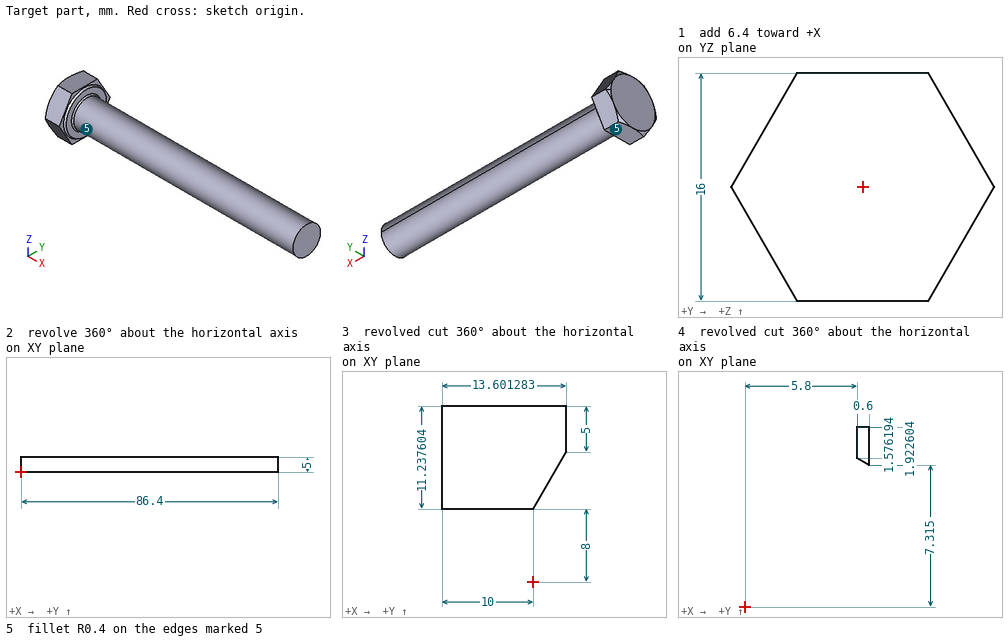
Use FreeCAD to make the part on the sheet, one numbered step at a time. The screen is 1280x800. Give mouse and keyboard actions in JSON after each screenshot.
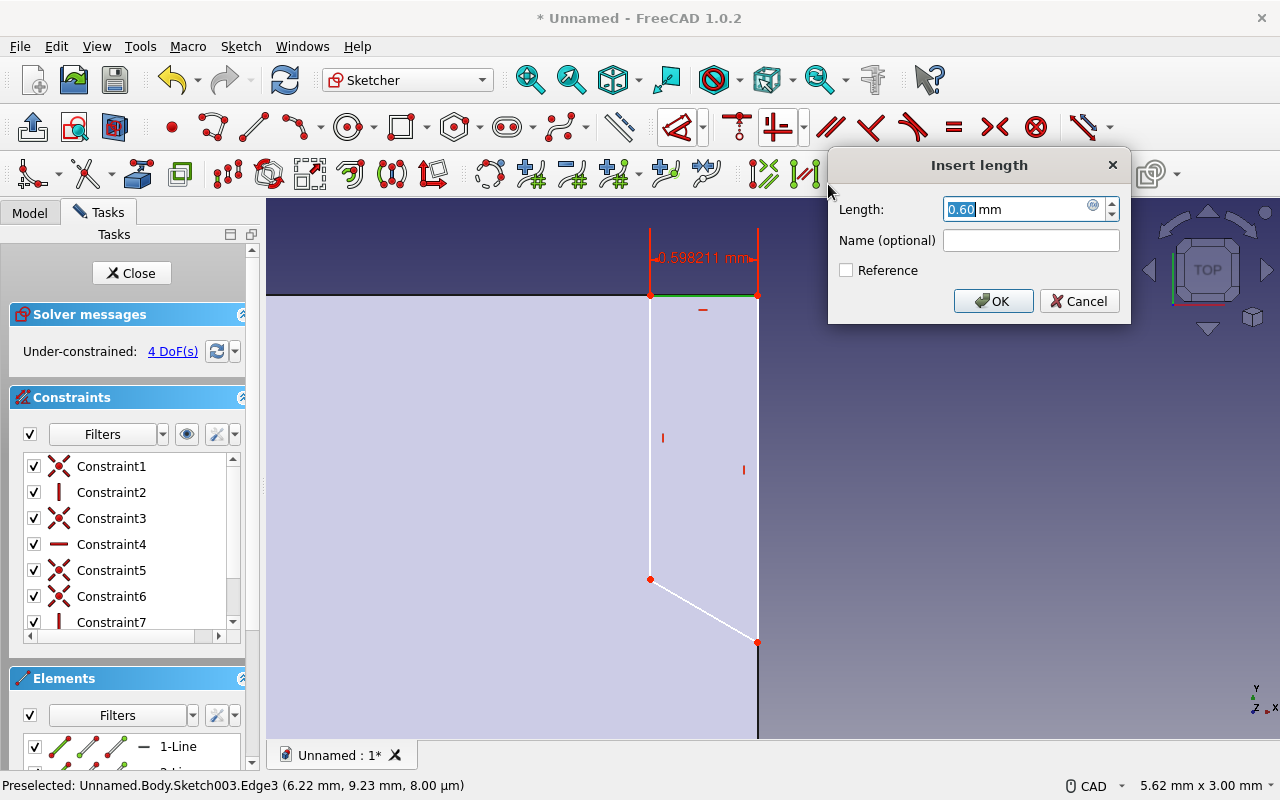
{"action": "type", "text": "0.6"}
{"action": "key", "text": "Return"}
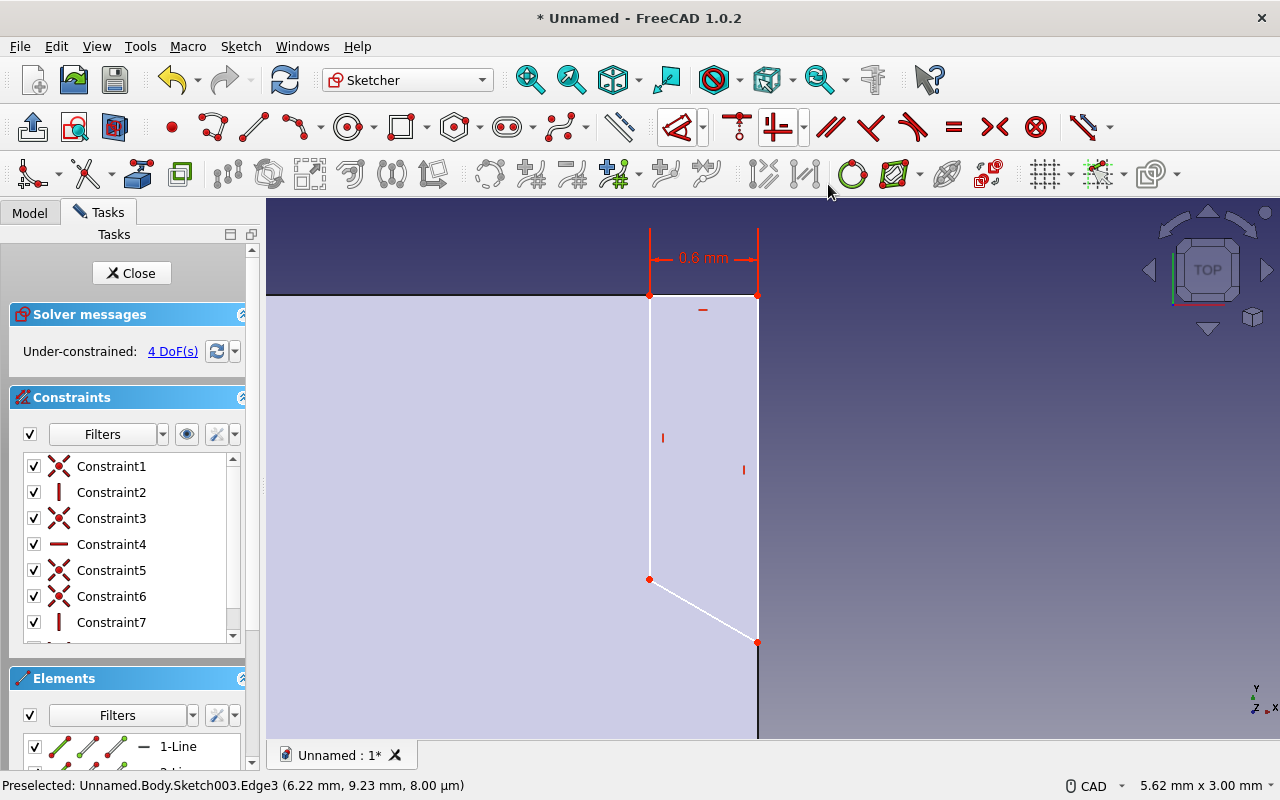
{"action": "left_click", "coordinate": [650, 580]}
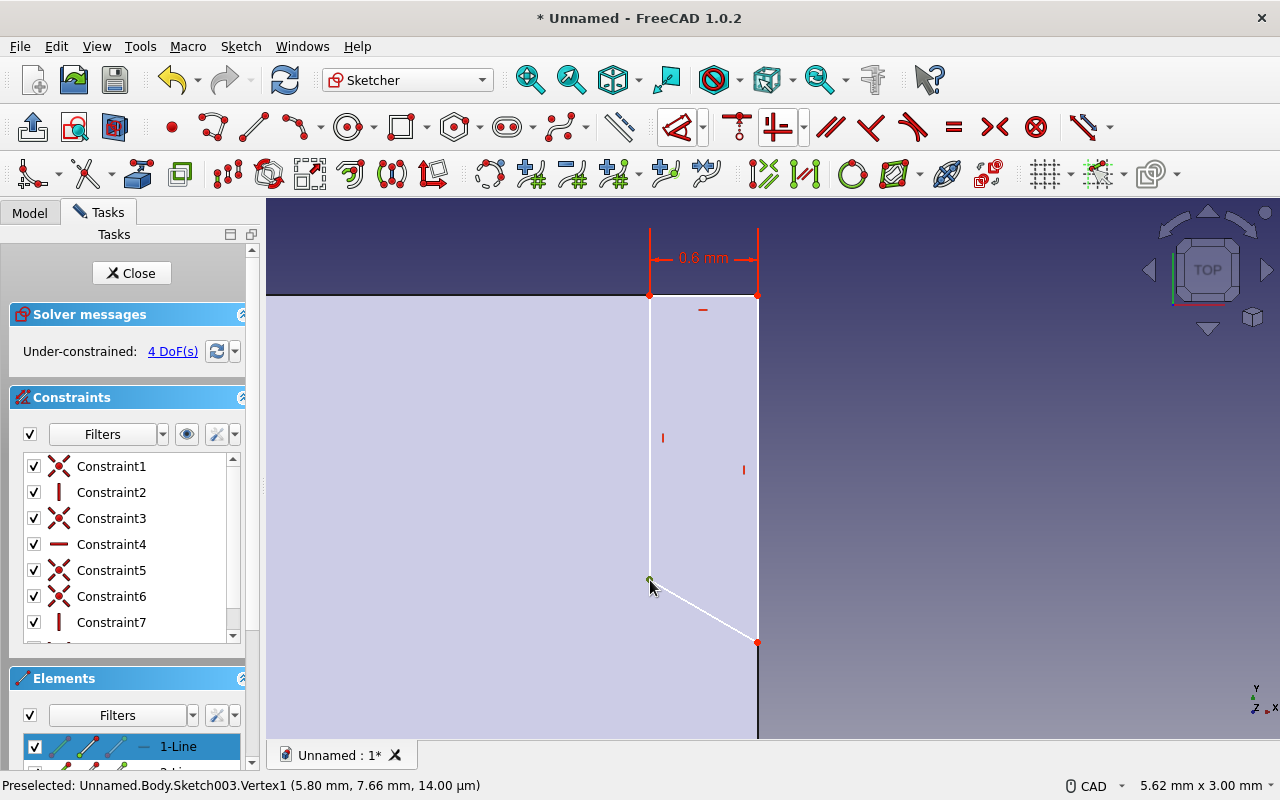
{"action": "key", "text": "l"}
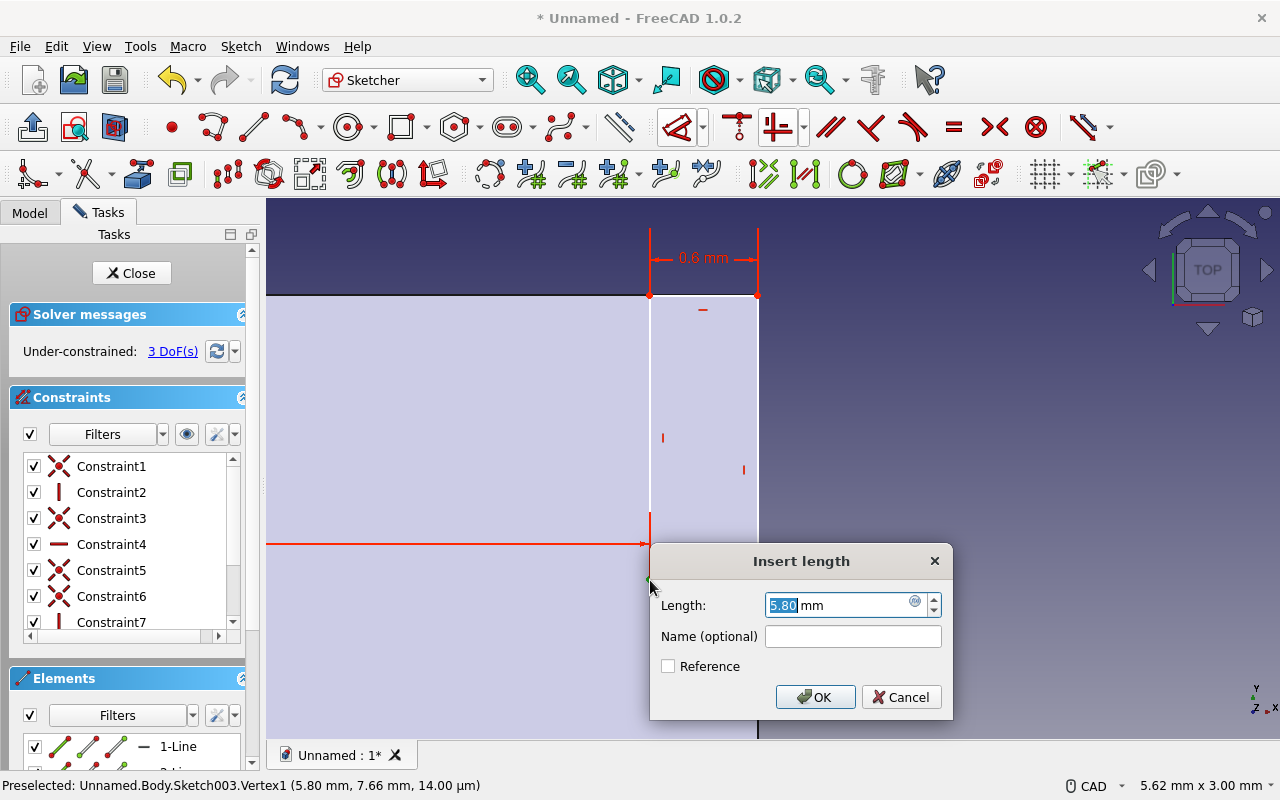
{"action": "type", "text": "5.8"}
{"action": "key", "text": "Return"}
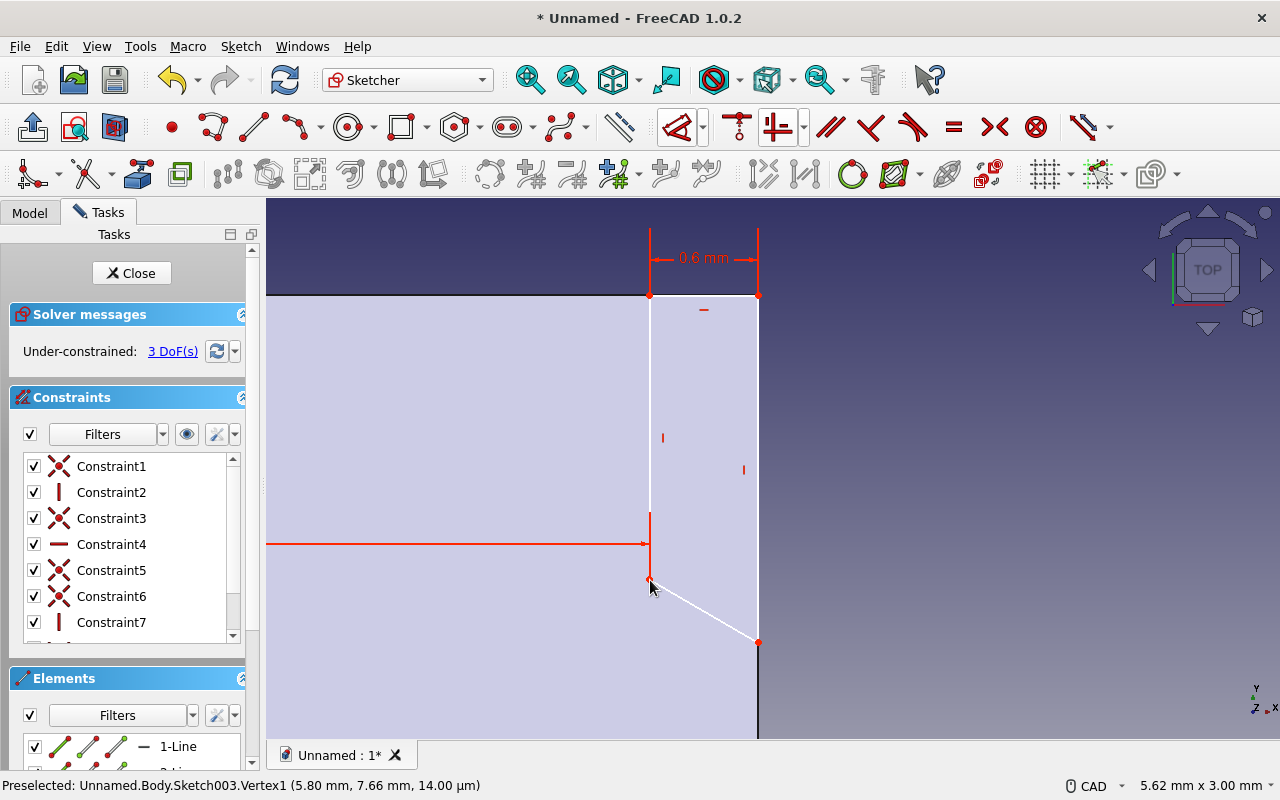
{"action": "left_click", "coordinate": [758, 643]}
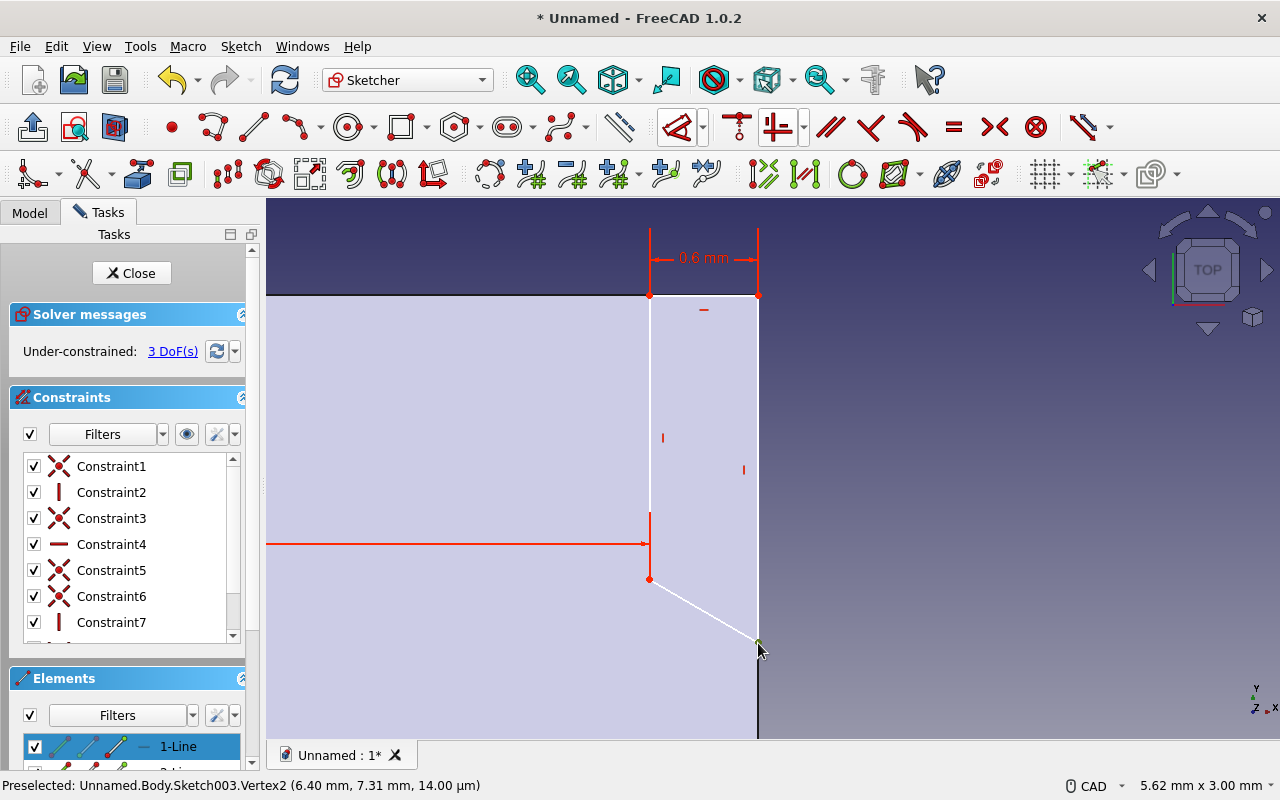
{"action": "key", "text": "i"}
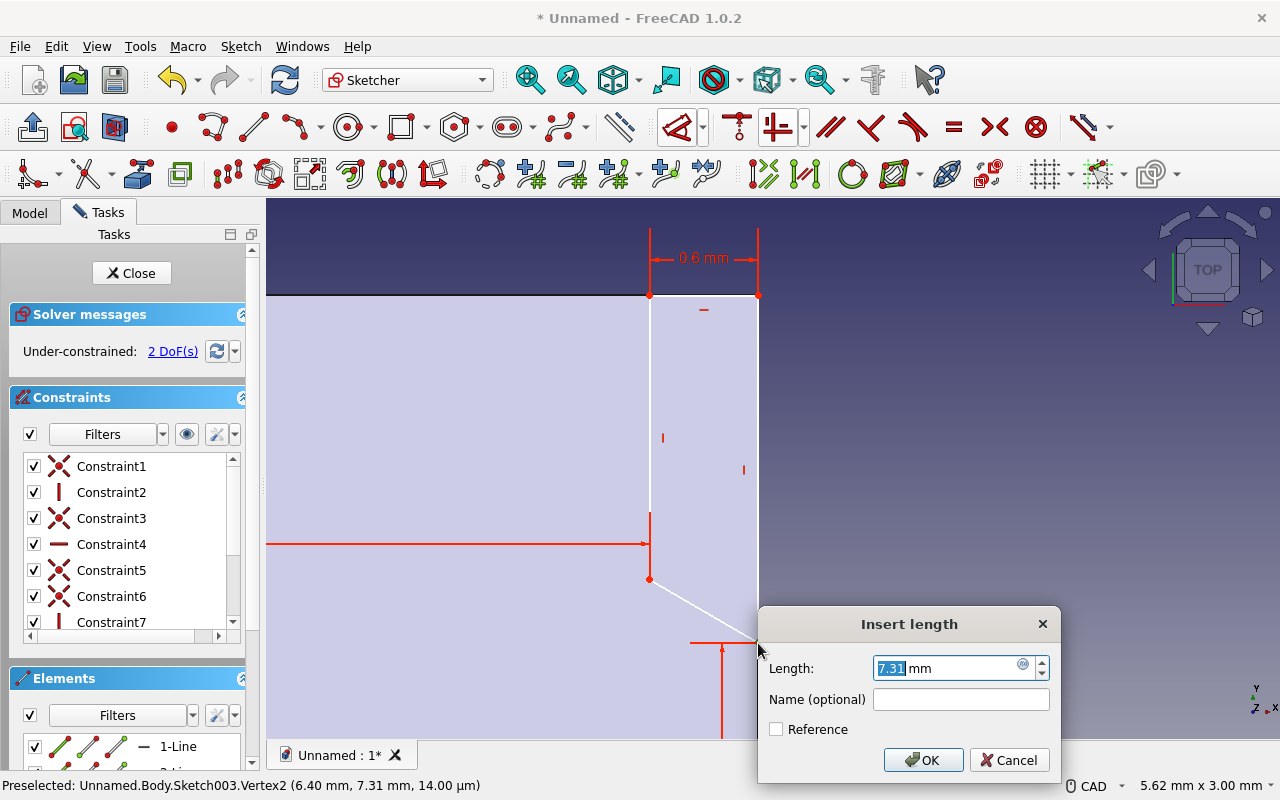
{"action": "type", "text": "7.315"}
{"action": "key", "text": "Return"}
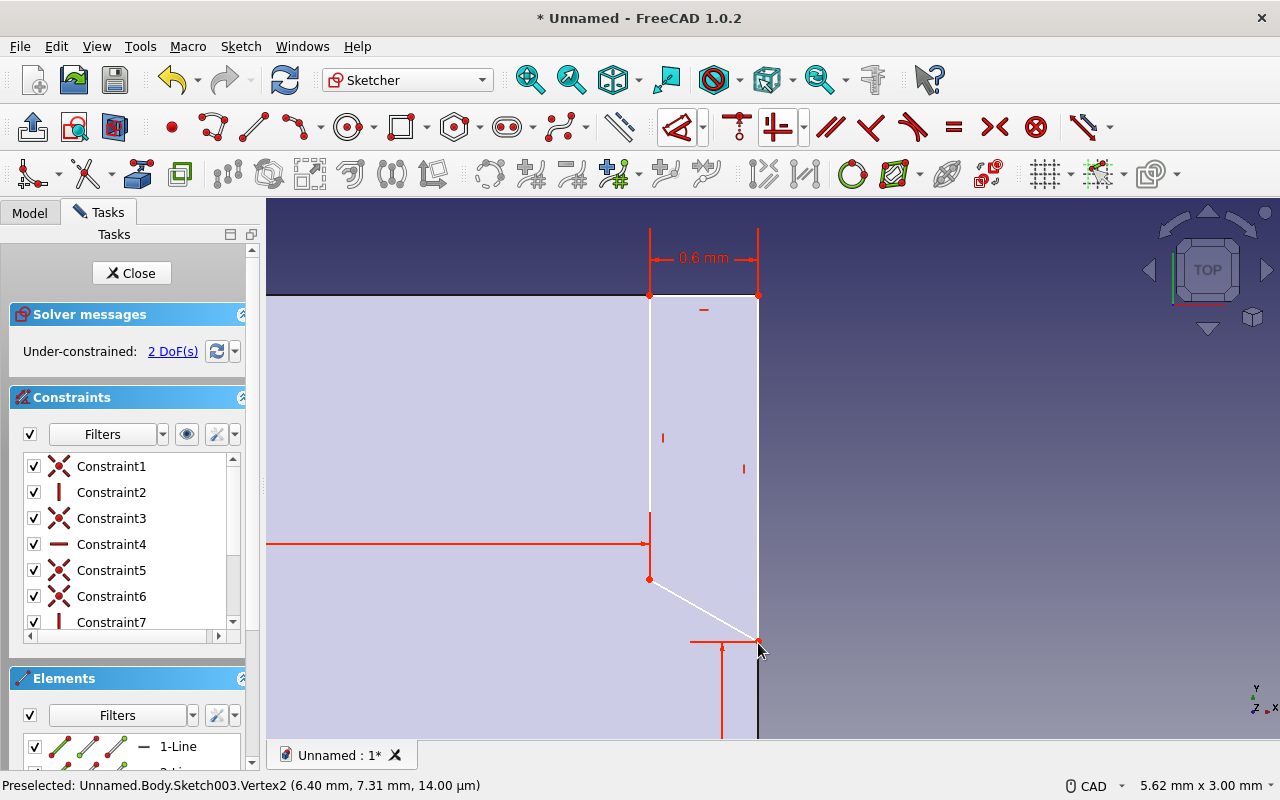
{"action": "left_click", "coordinate": [758, 538]}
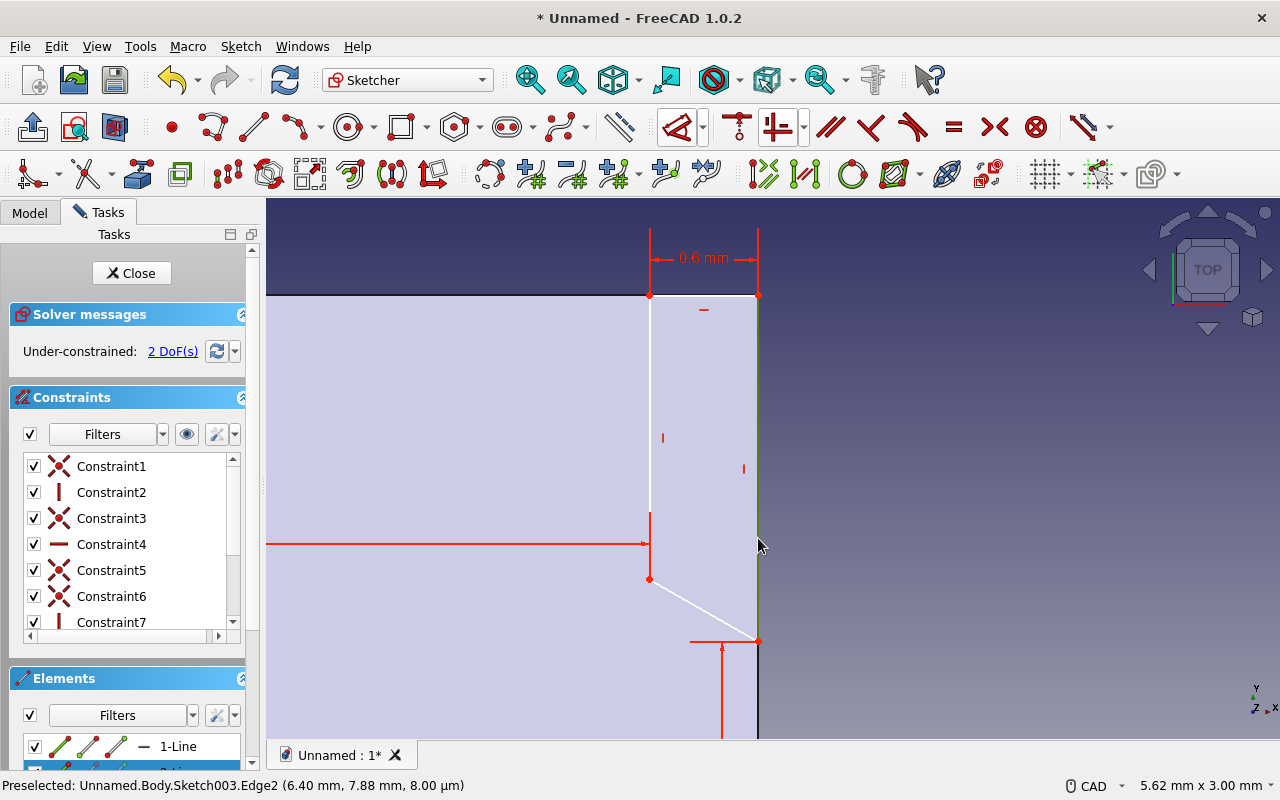
{"action": "left_click", "coordinate": [702, 128]}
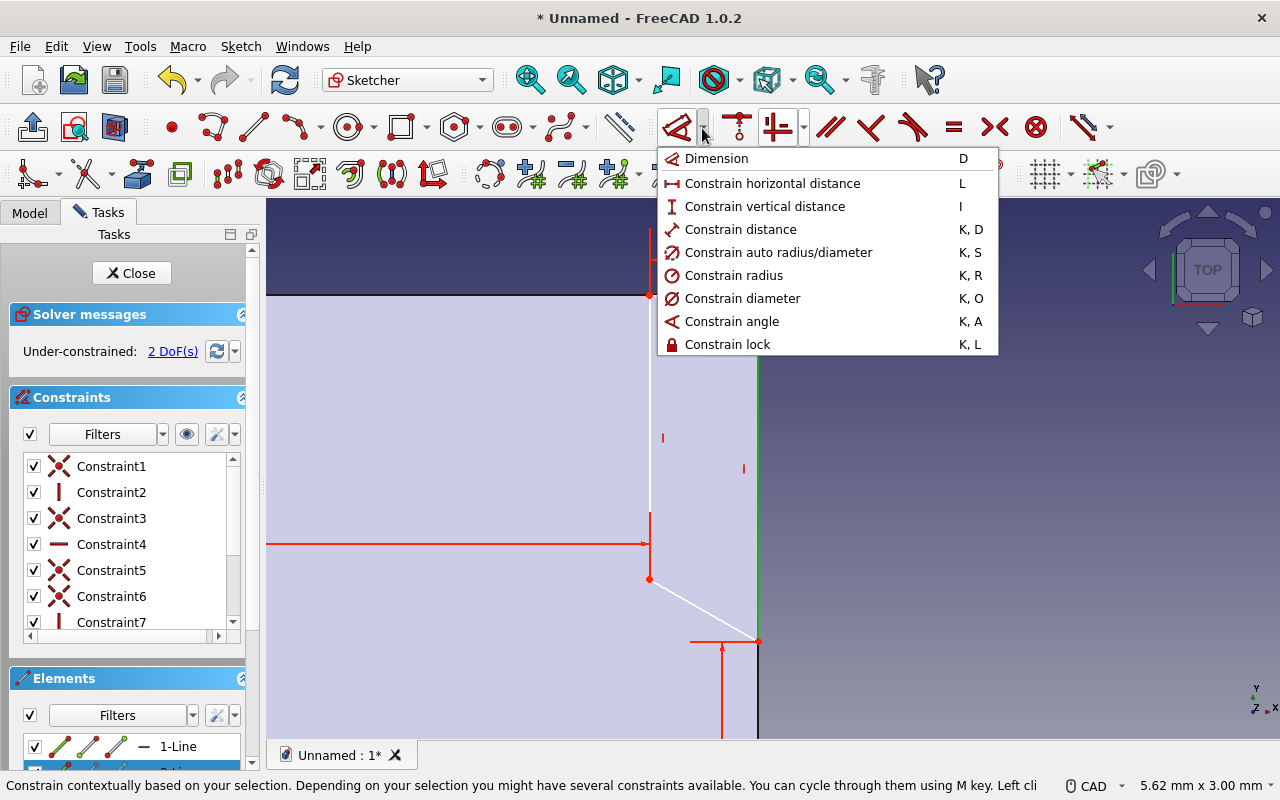
{"action": "left_click", "coordinate": [828, 206]}